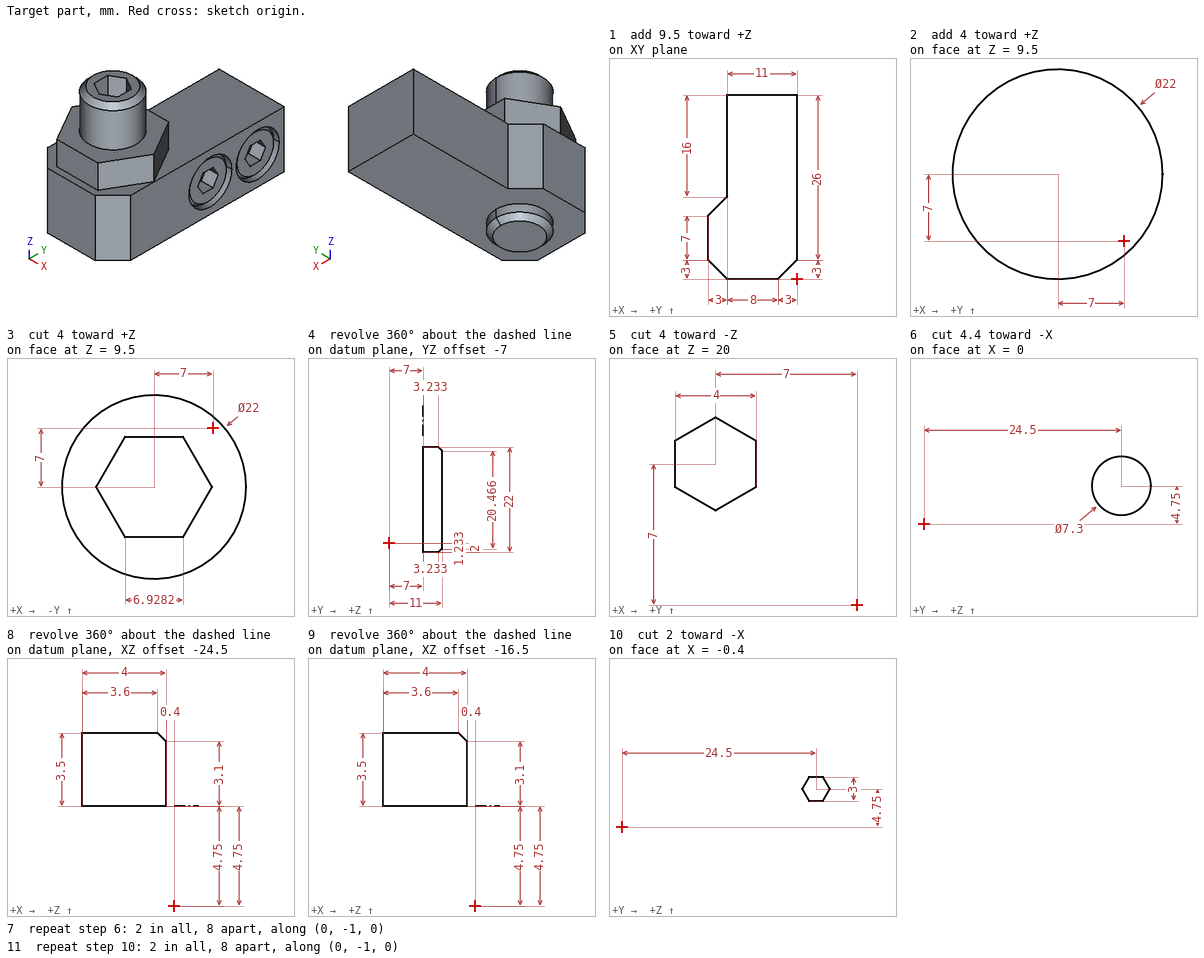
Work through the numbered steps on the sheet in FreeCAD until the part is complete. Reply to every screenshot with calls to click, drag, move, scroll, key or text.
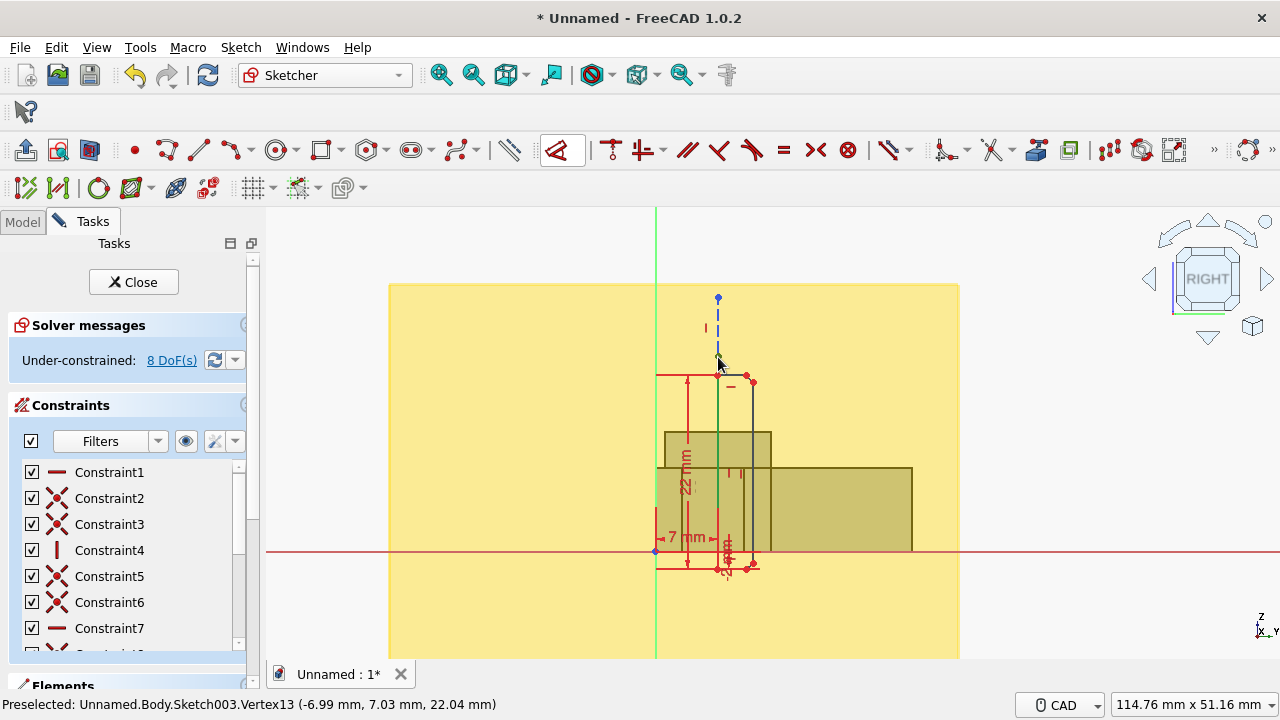
key(l)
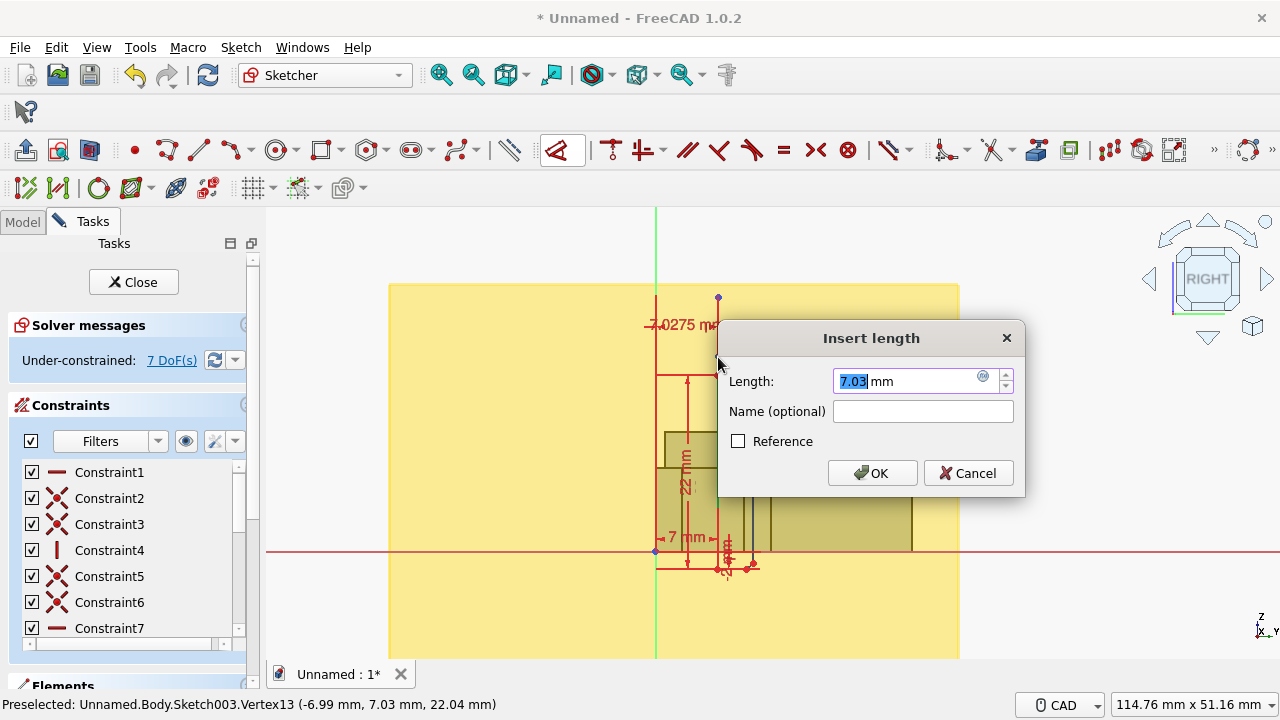
text(7)
key(Return)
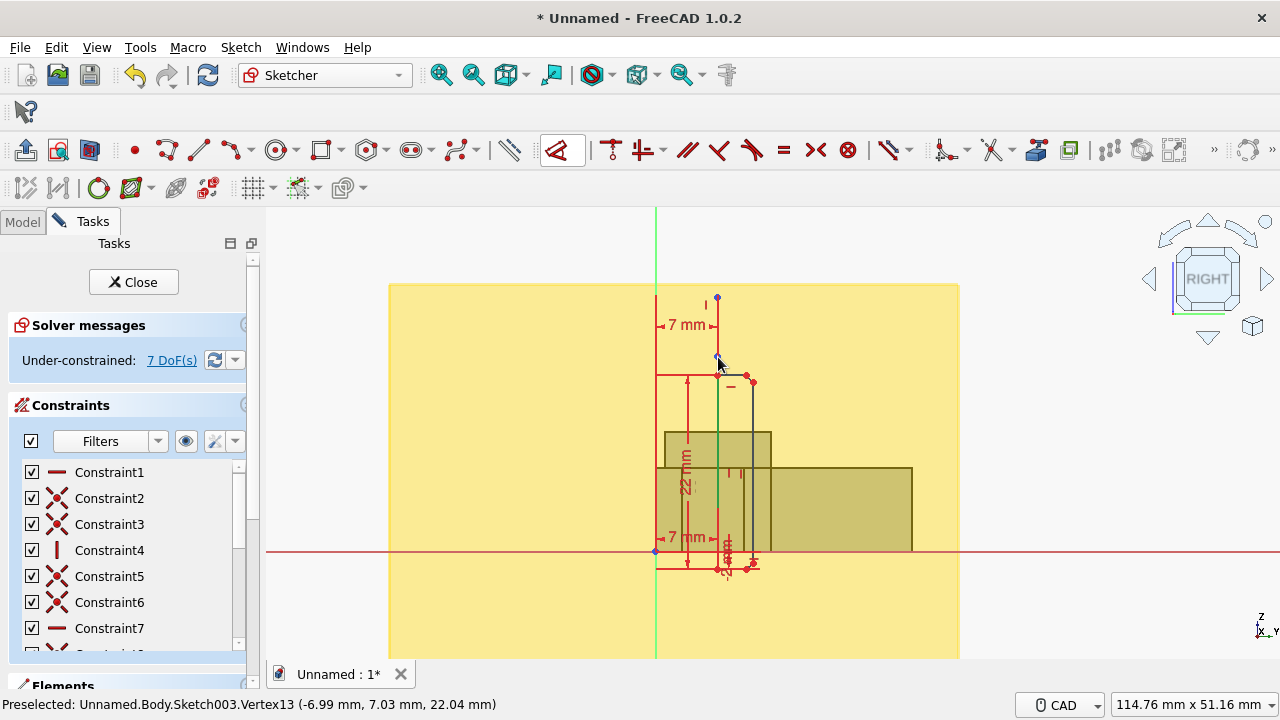
scroll(753, 563, up, 2)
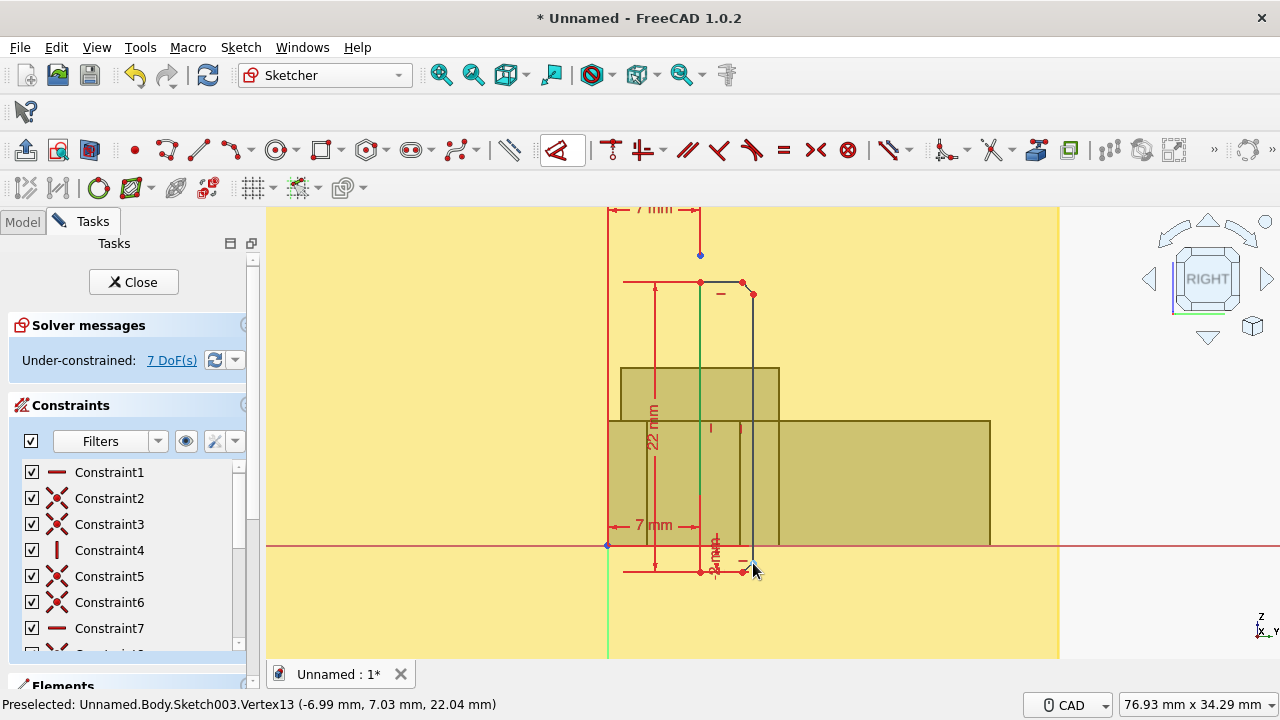
click(753, 563)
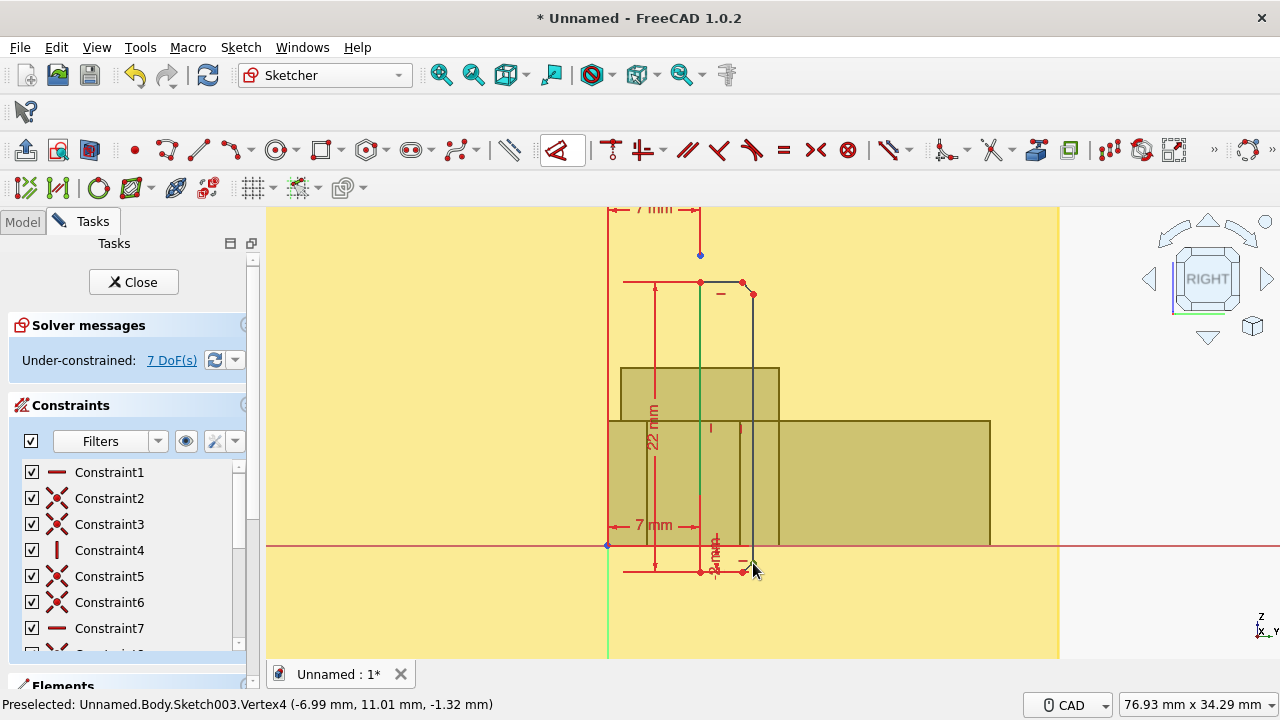
click(580, 150)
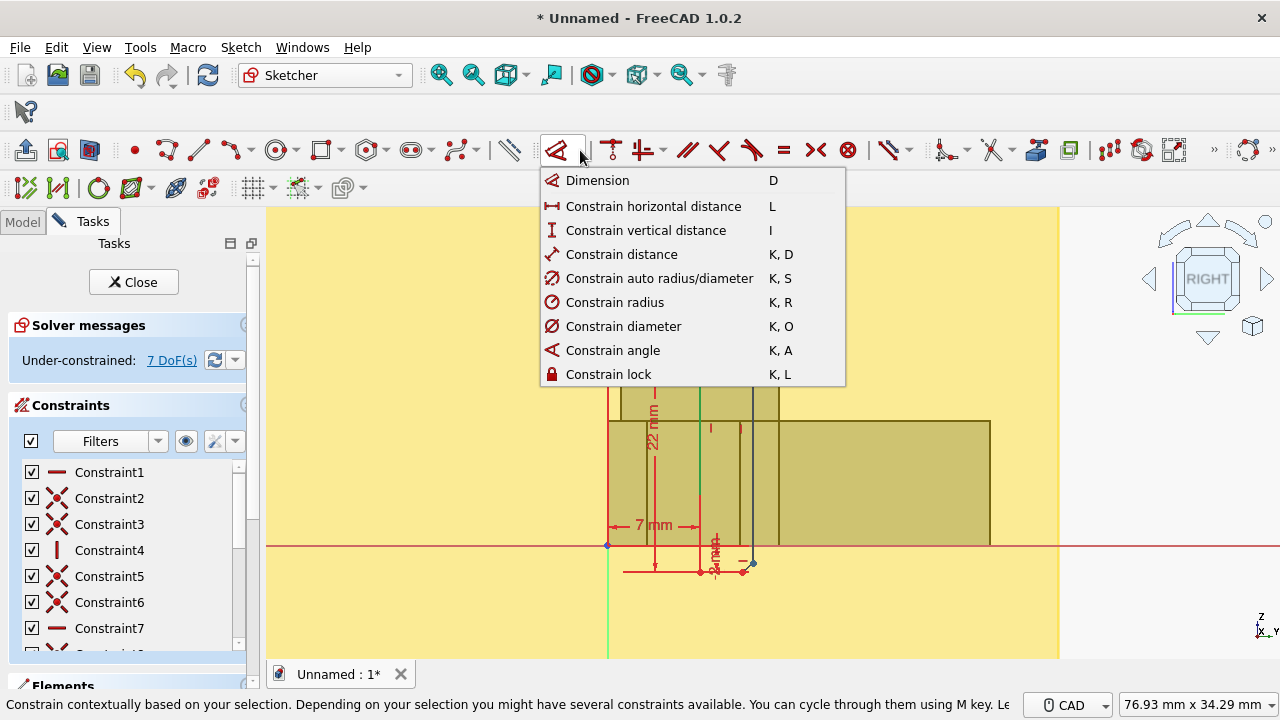
click(693, 206)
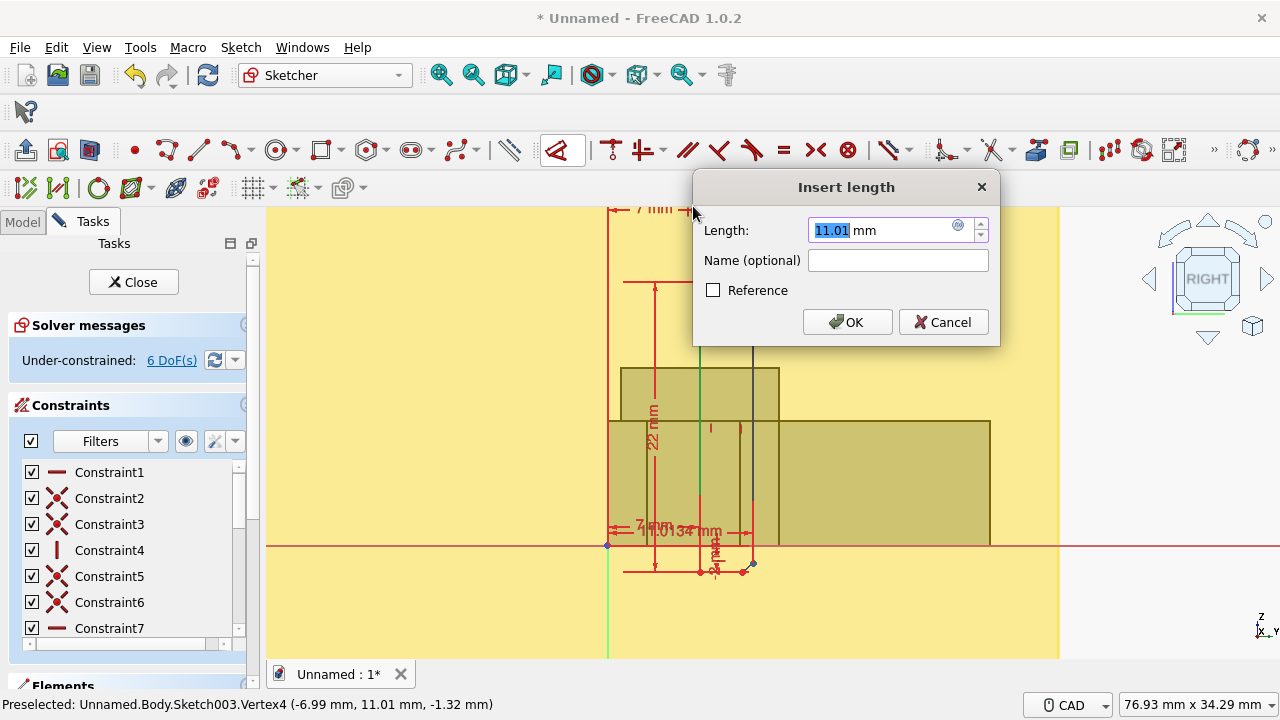
text(11)
key(Return)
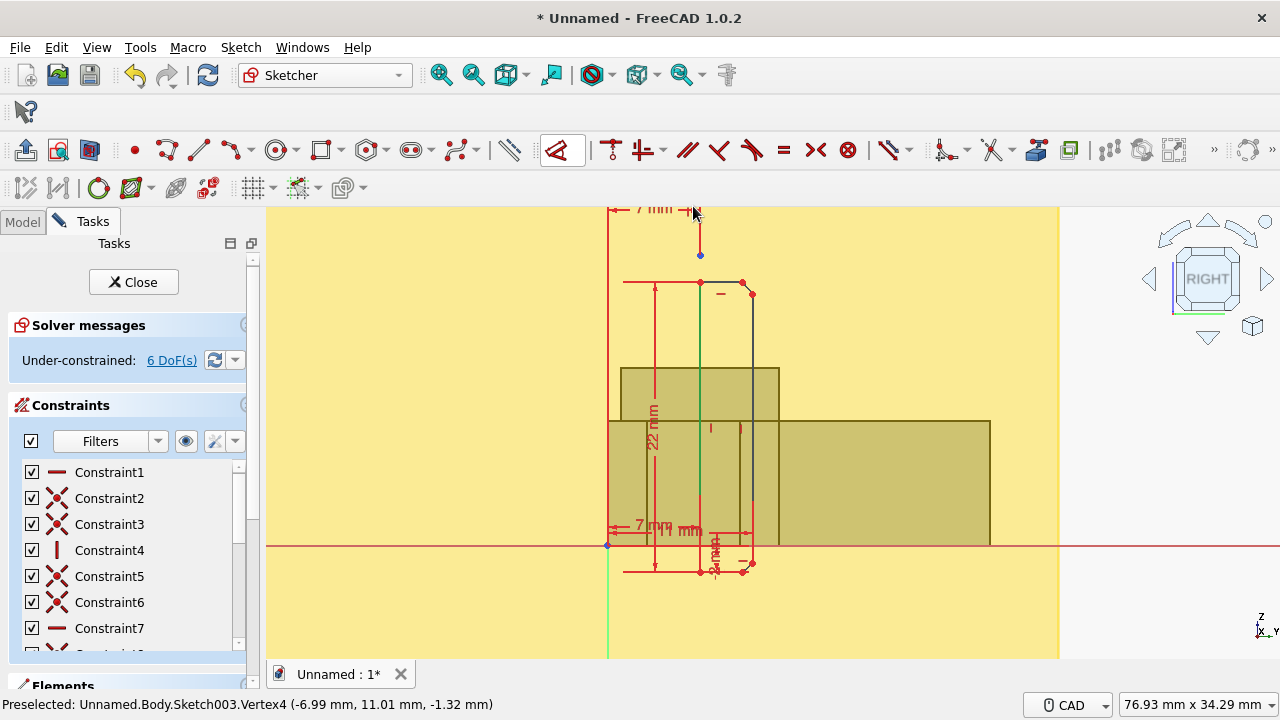
click(730, 572)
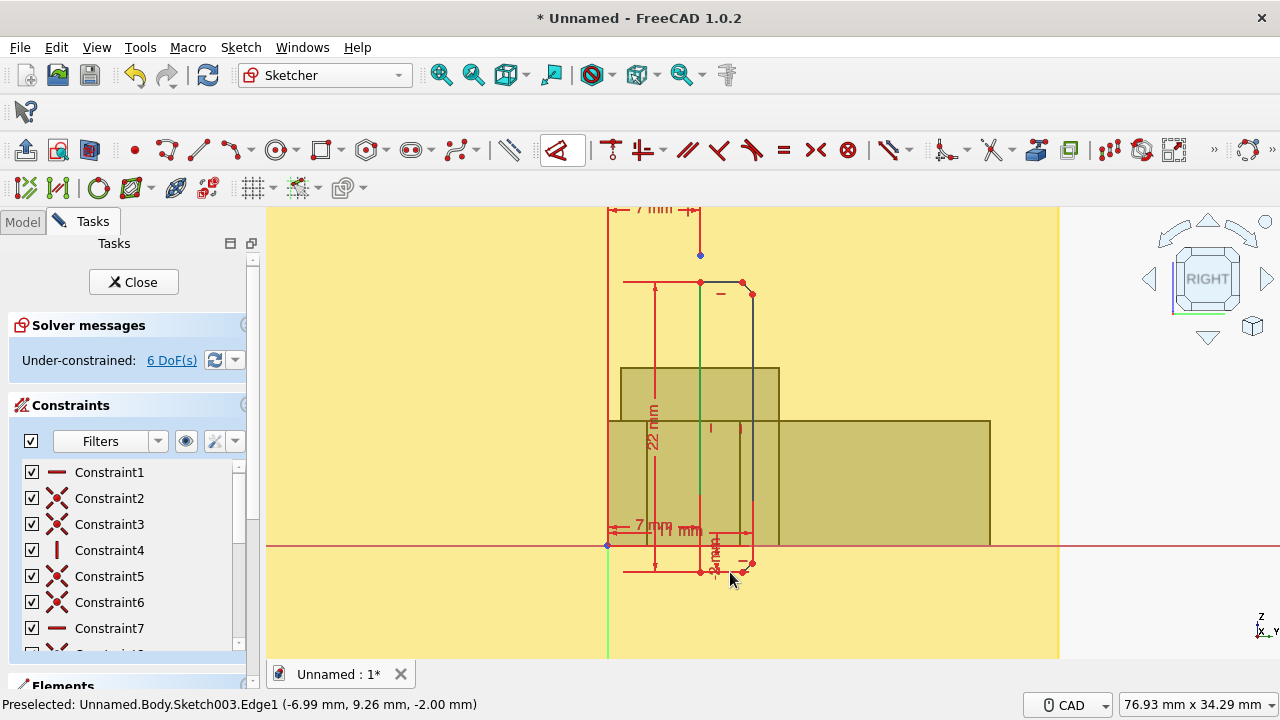
key(l)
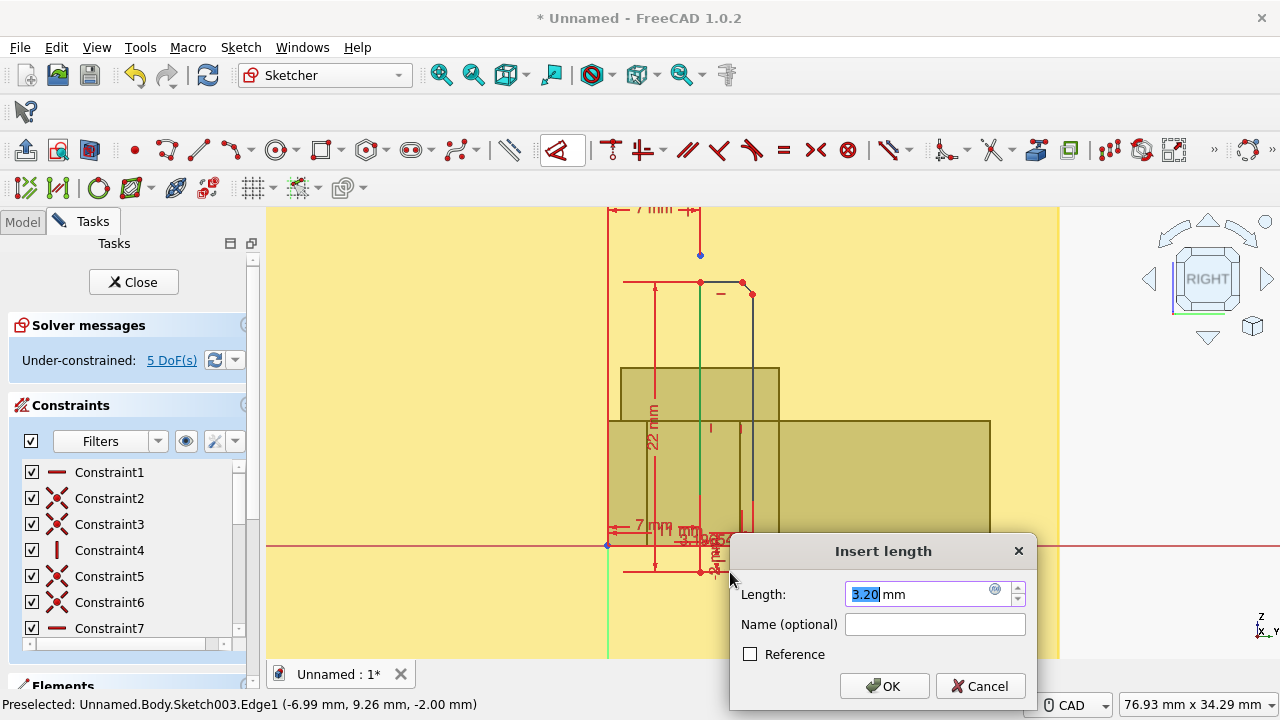
text(3.233)
key(Return)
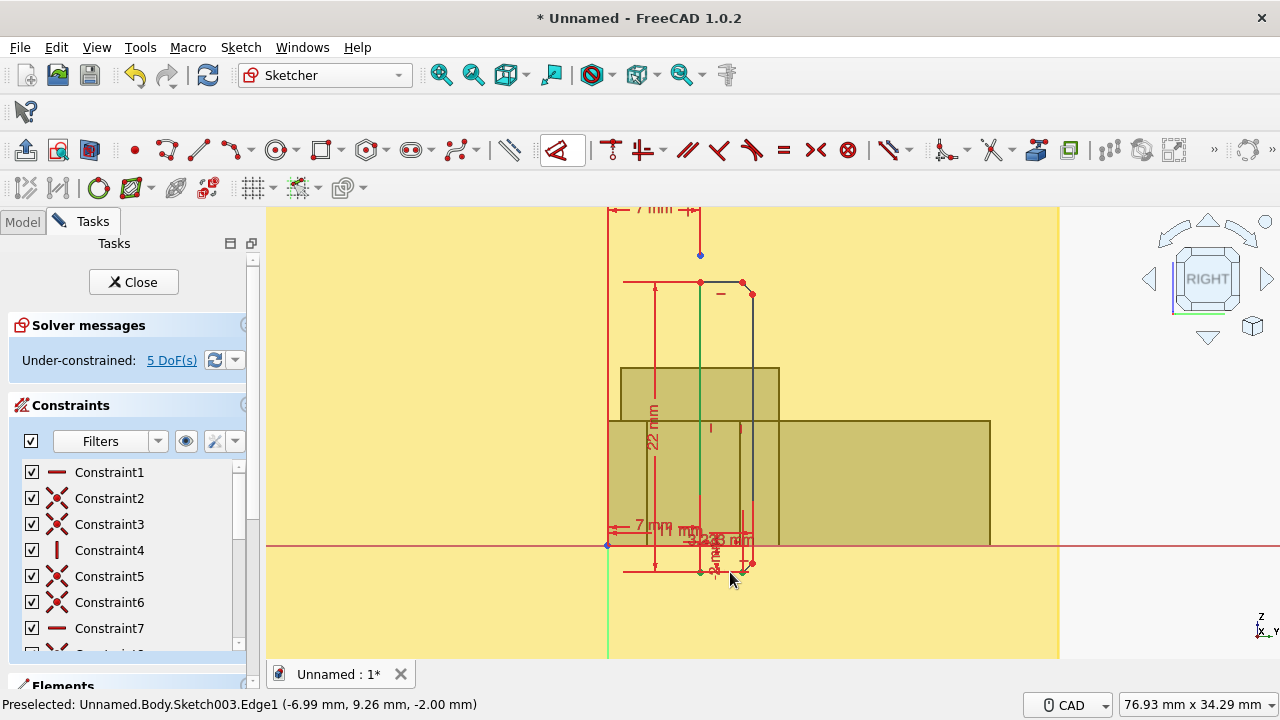
click(730, 282)